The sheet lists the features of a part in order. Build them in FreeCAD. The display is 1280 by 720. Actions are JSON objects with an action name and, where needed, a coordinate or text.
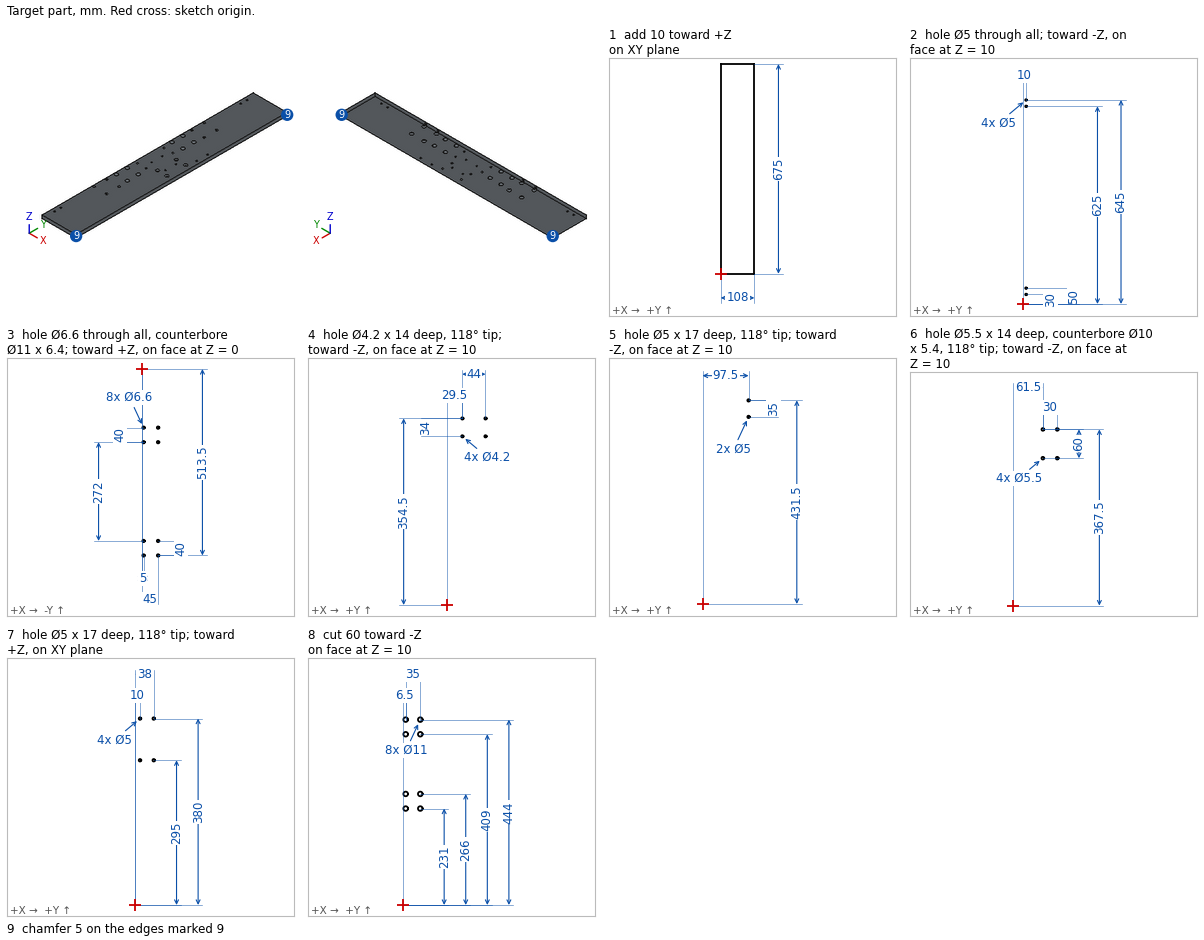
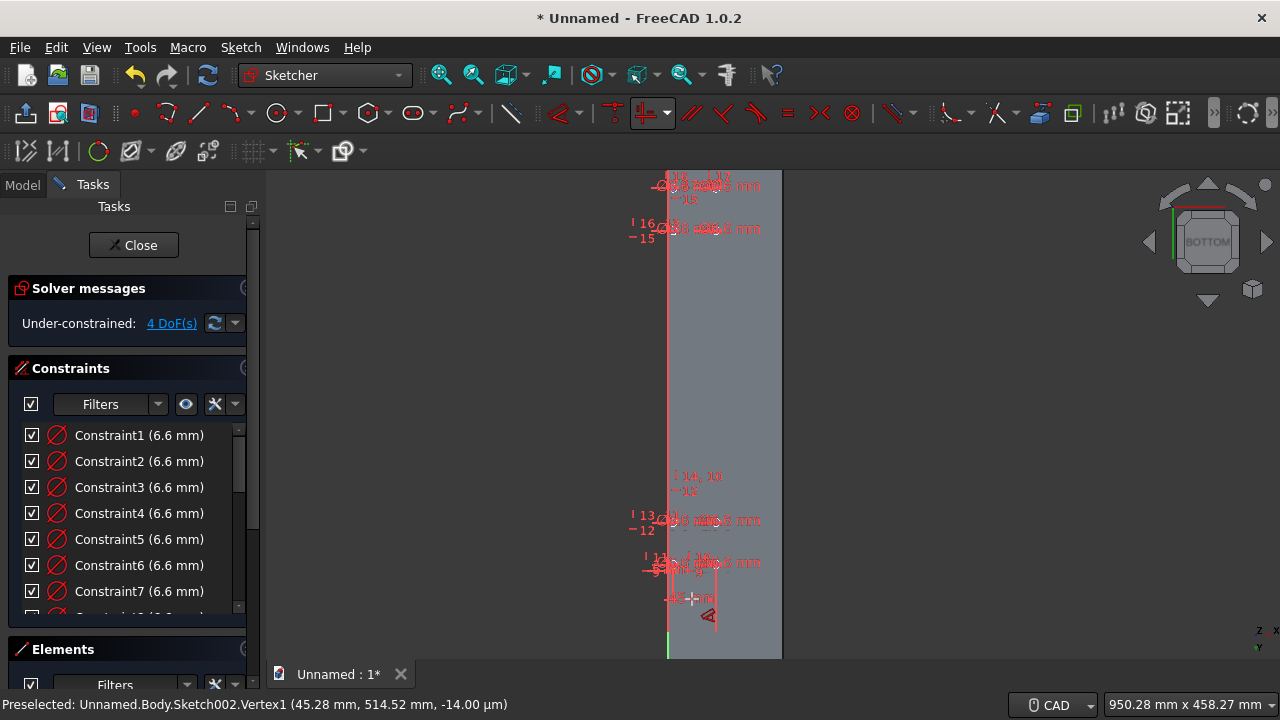
{"action": "left_click", "coordinate": [716, 565]}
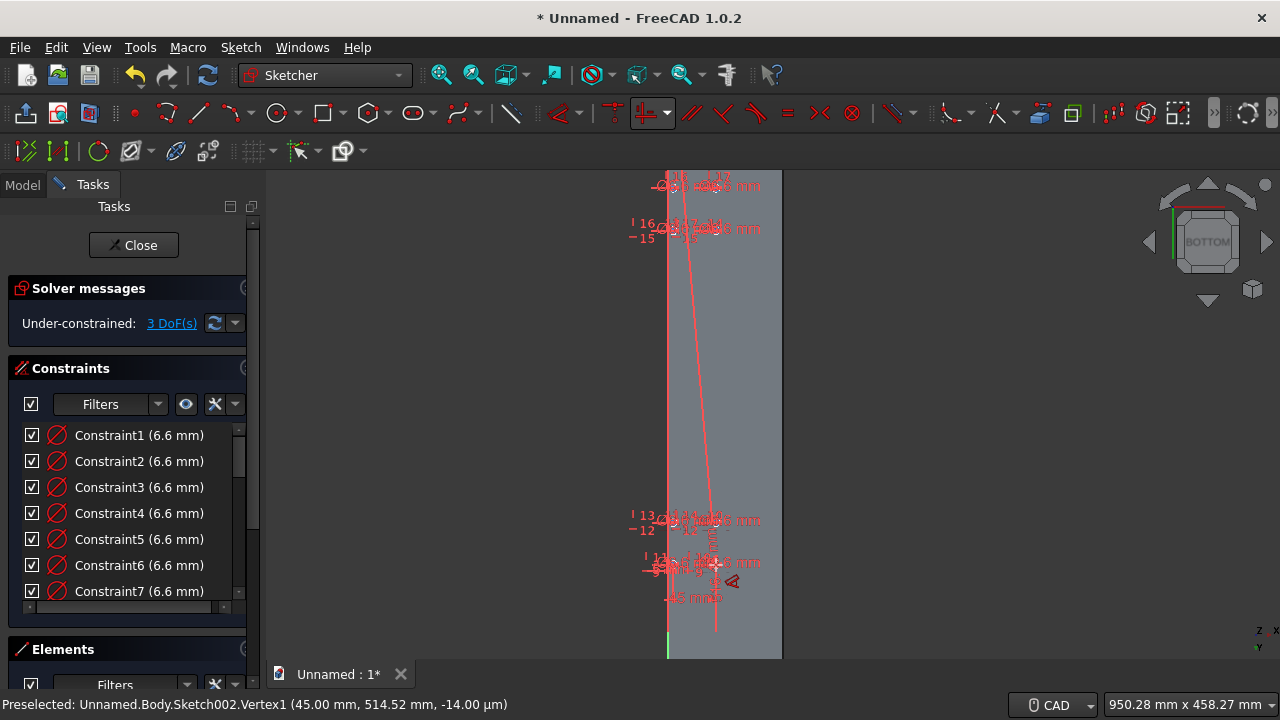
{"action": "left_click", "coordinate": [716, 523]}
{"action": "left_click", "coordinate": [750, 544]}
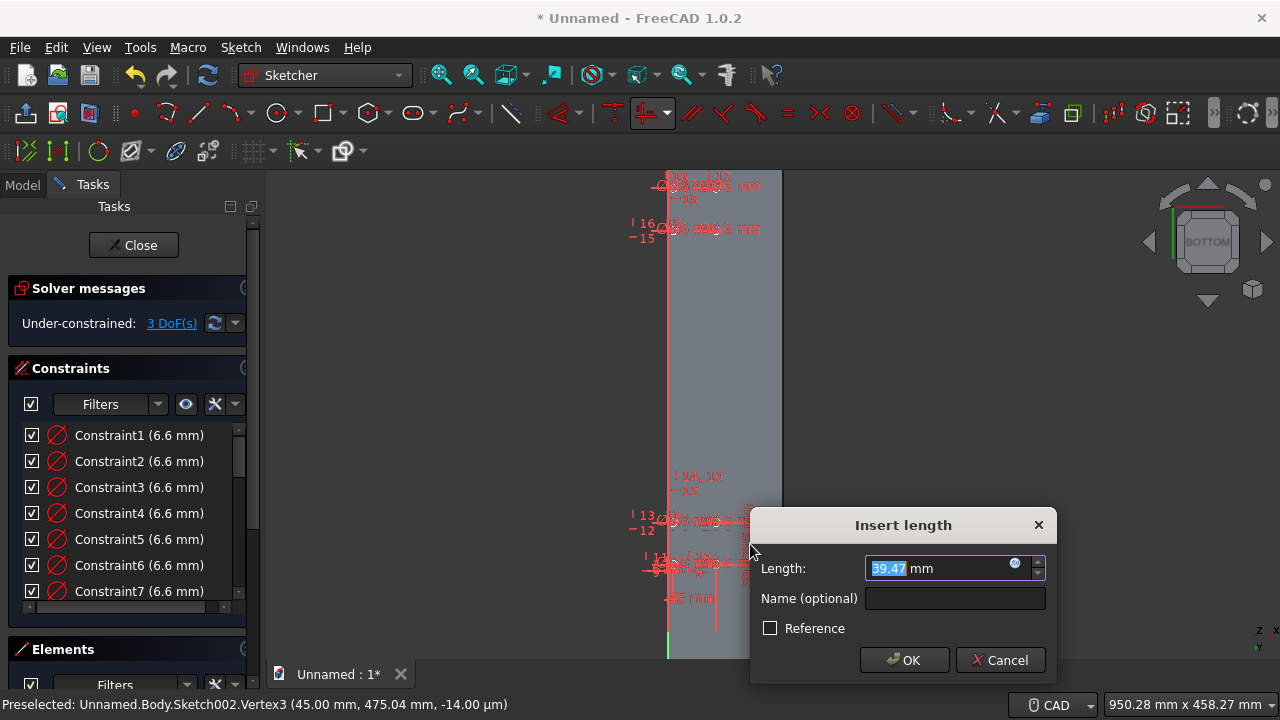
{"action": "type", "text": "40"}
{"action": "key", "text": "Return"}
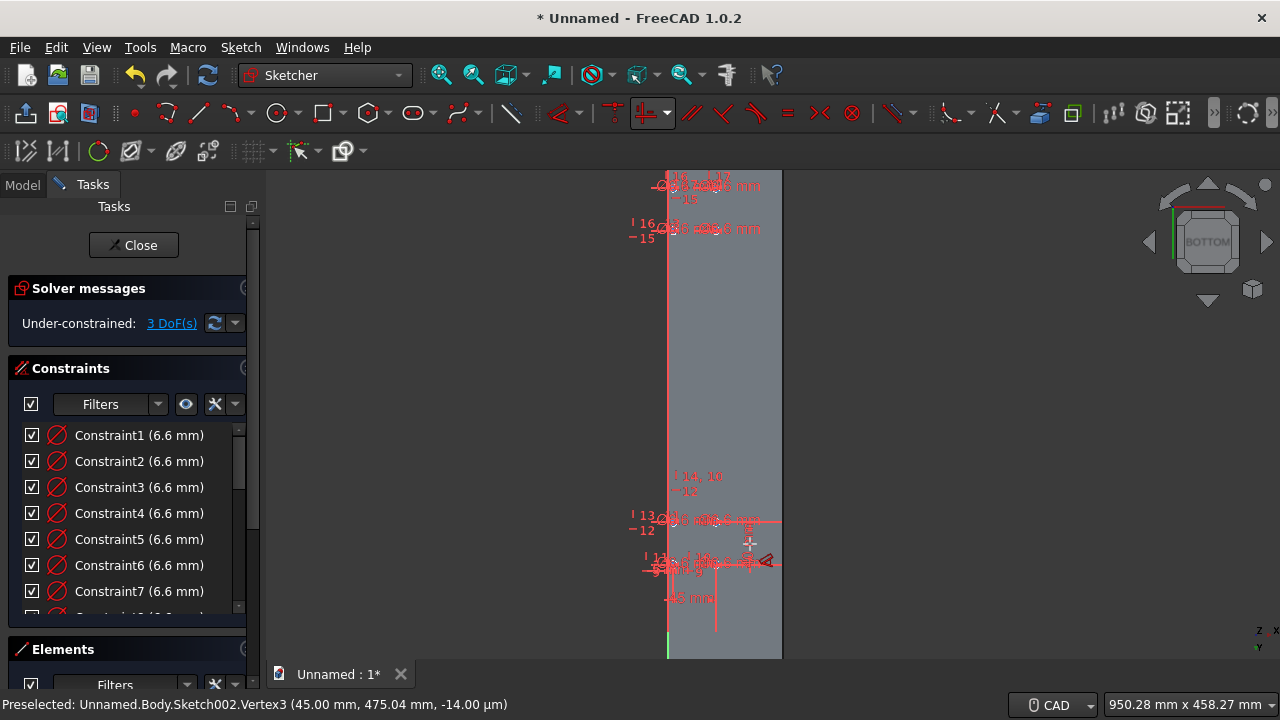
{"action": "left_click", "coordinate": [673, 231]}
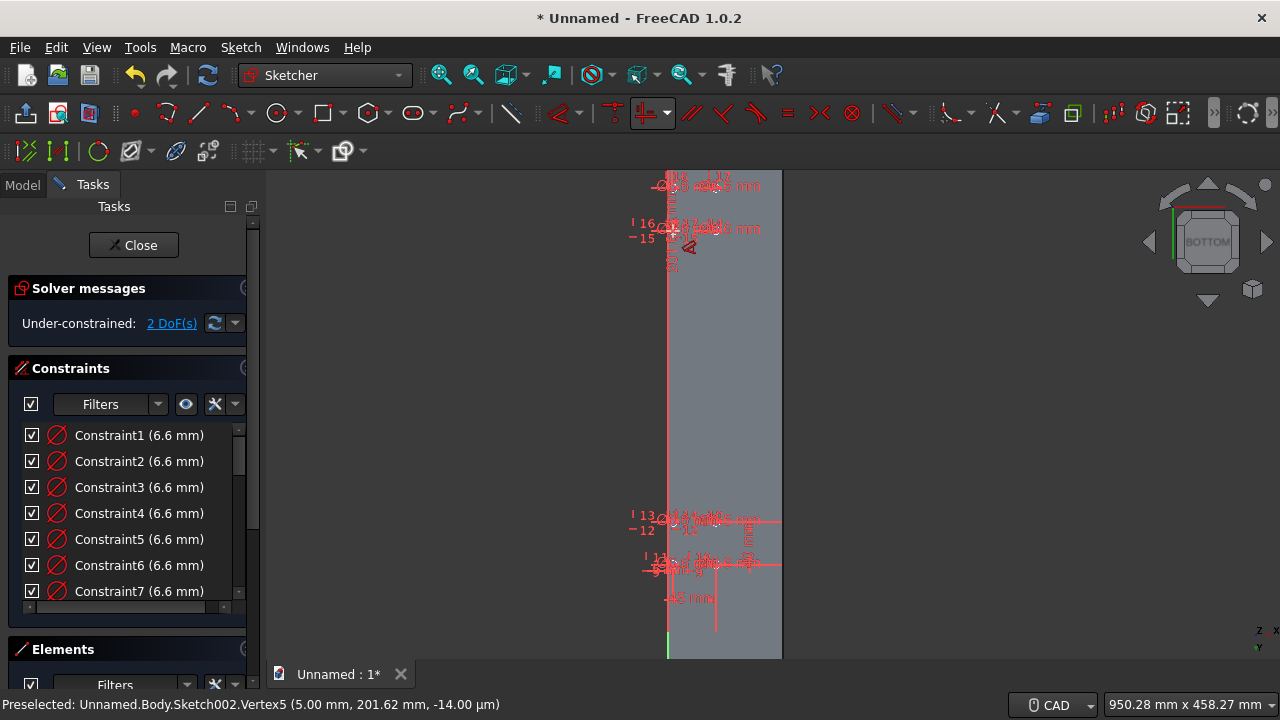
{"action": "scroll", "coordinate": [717, 564], "scroll_direction": "down", "scroll_amount": 3}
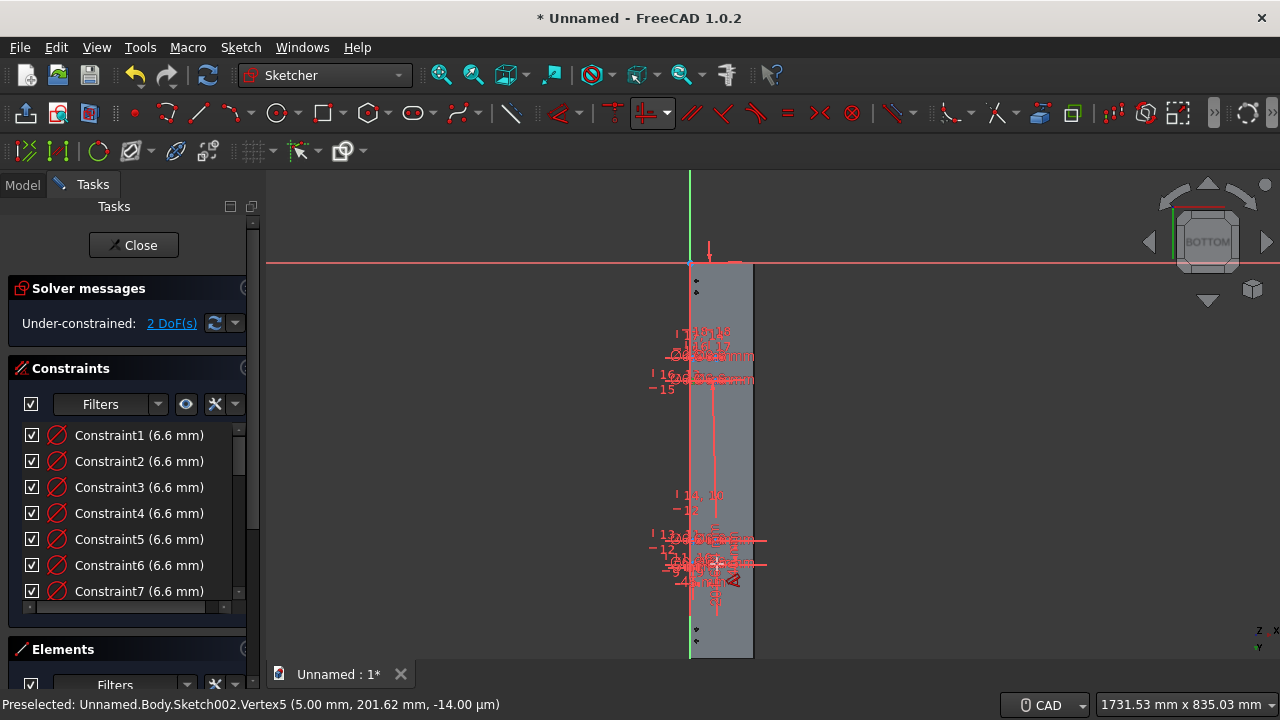
{"action": "scroll", "coordinate": [693, 358], "scroll_direction": "up", "scroll_amount": 3}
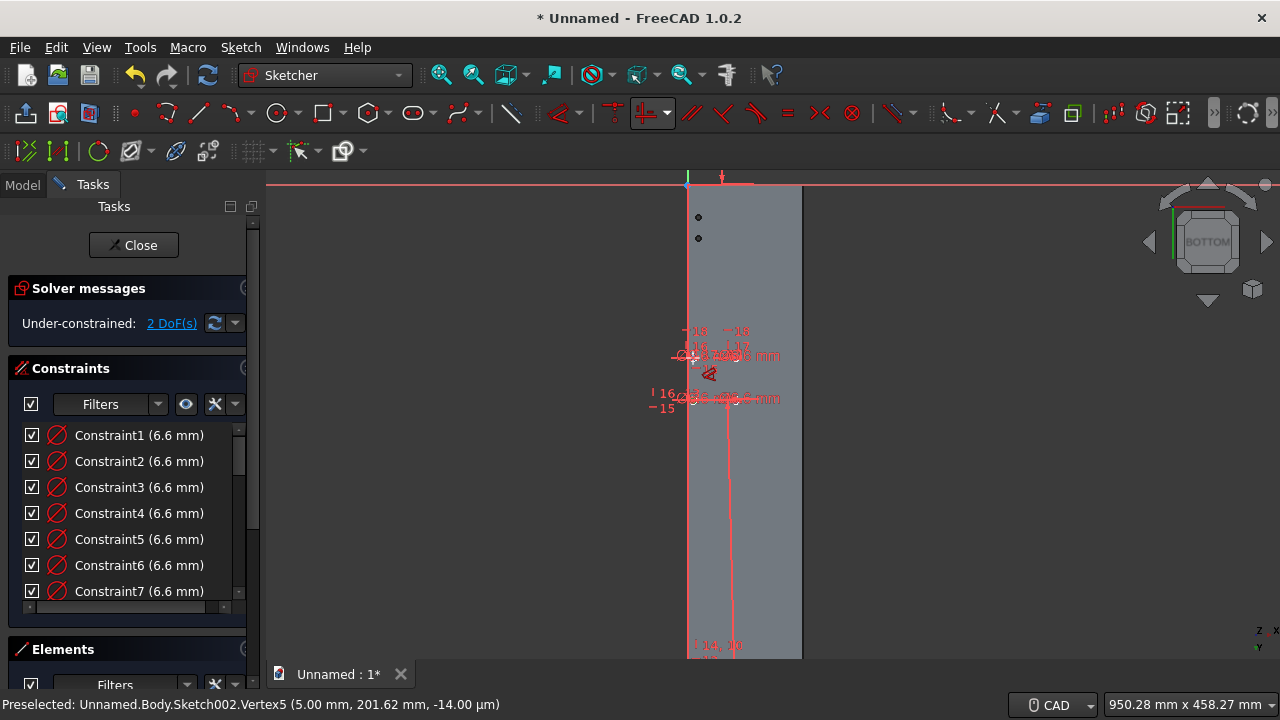
{"action": "left_click", "coordinate": [693, 358]}
{"action": "left_click", "coordinate": [659, 379]}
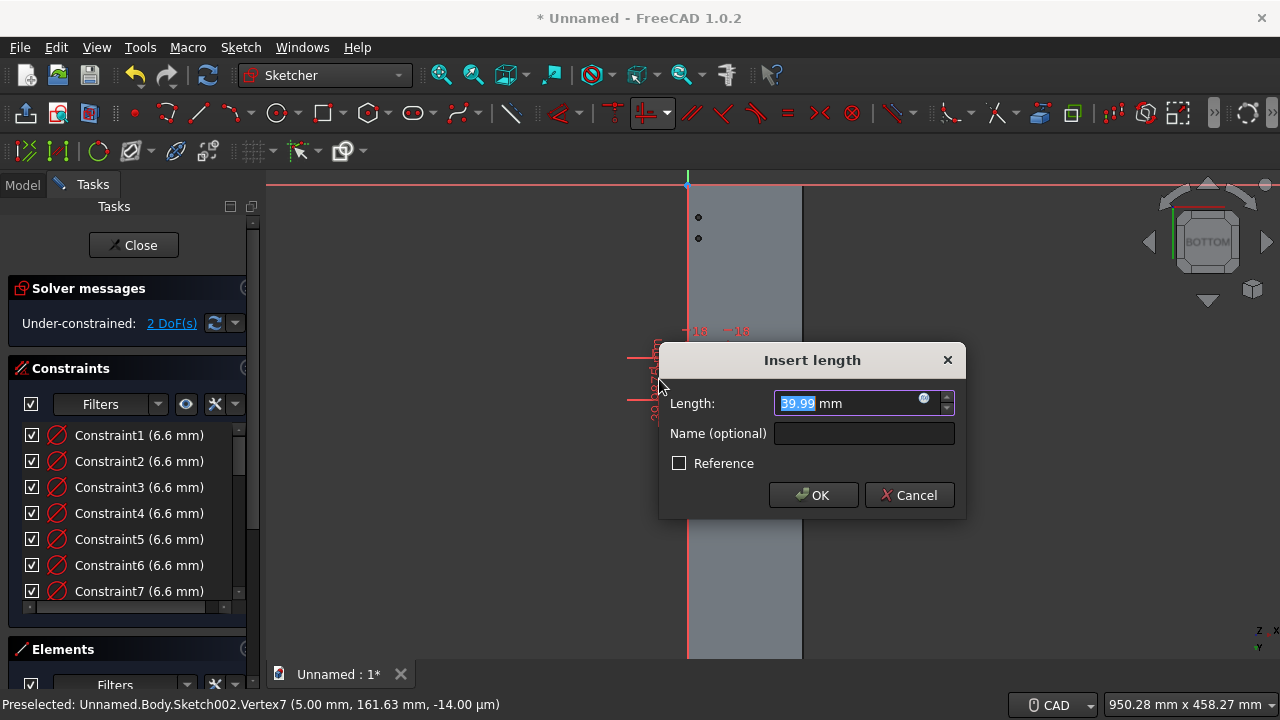
{"action": "type", "text": "40"}
{"action": "key", "text": "Return"}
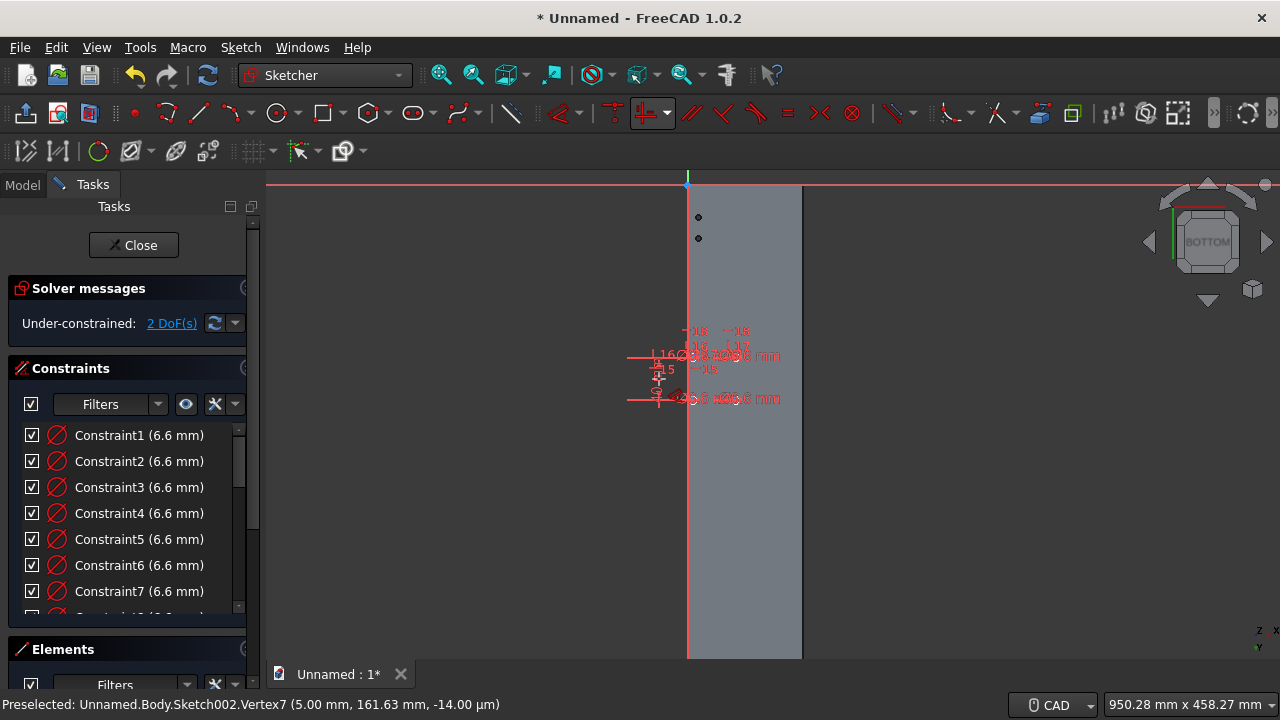
{"action": "scroll", "coordinate": [693, 358], "scroll_direction": "down", "scroll_amount": 3}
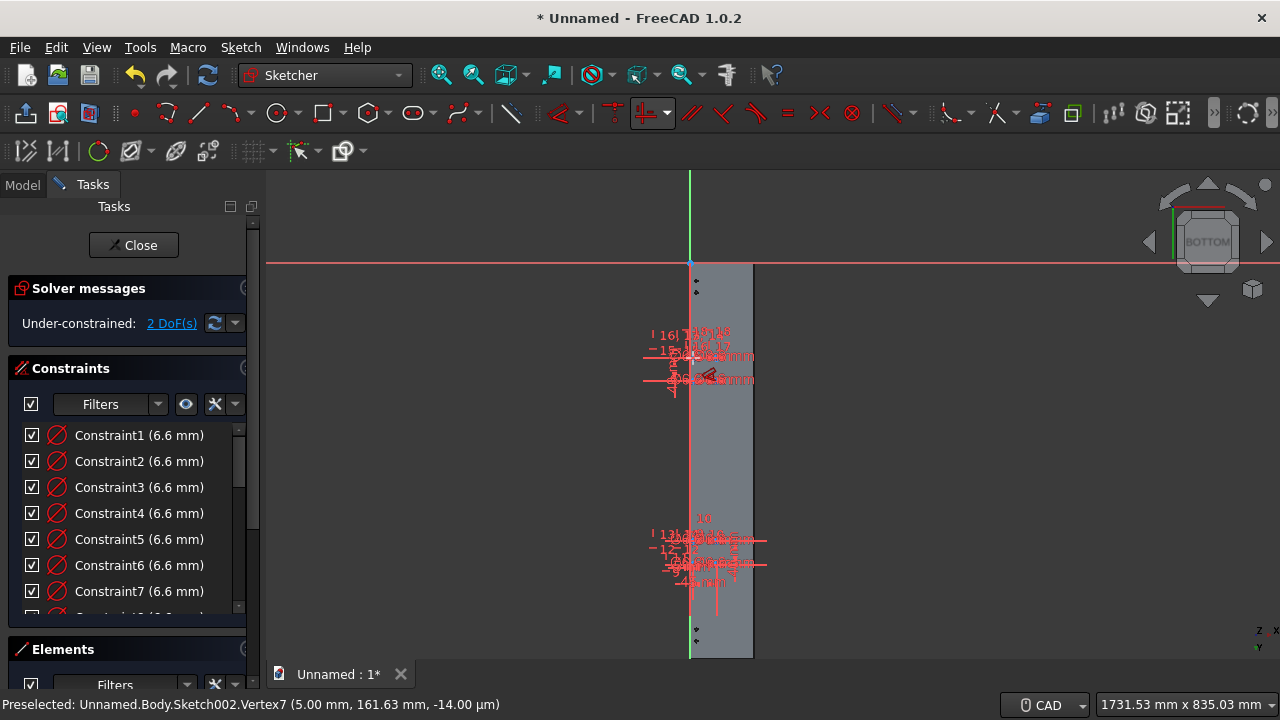
{"action": "left_click", "coordinate": [693, 541]}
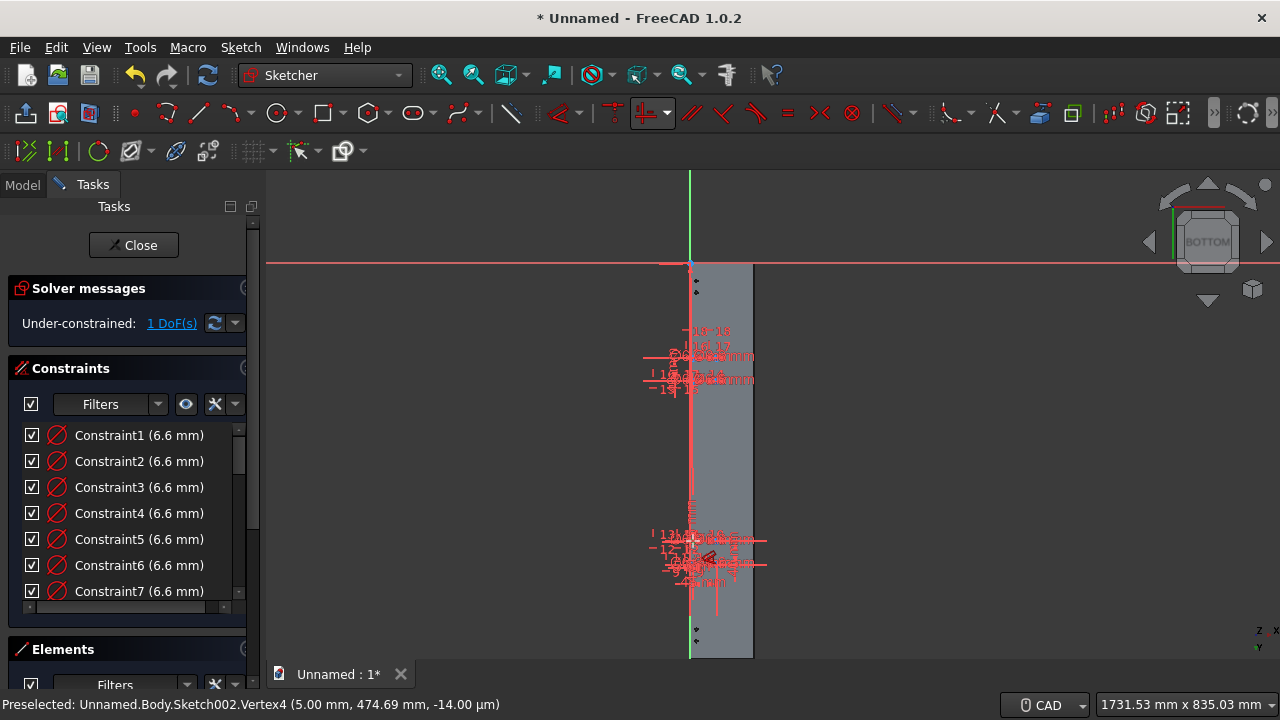
{"action": "left_click", "coordinate": [693, 381]}
{"action": "left_click", "coordinate": [659, 461]}